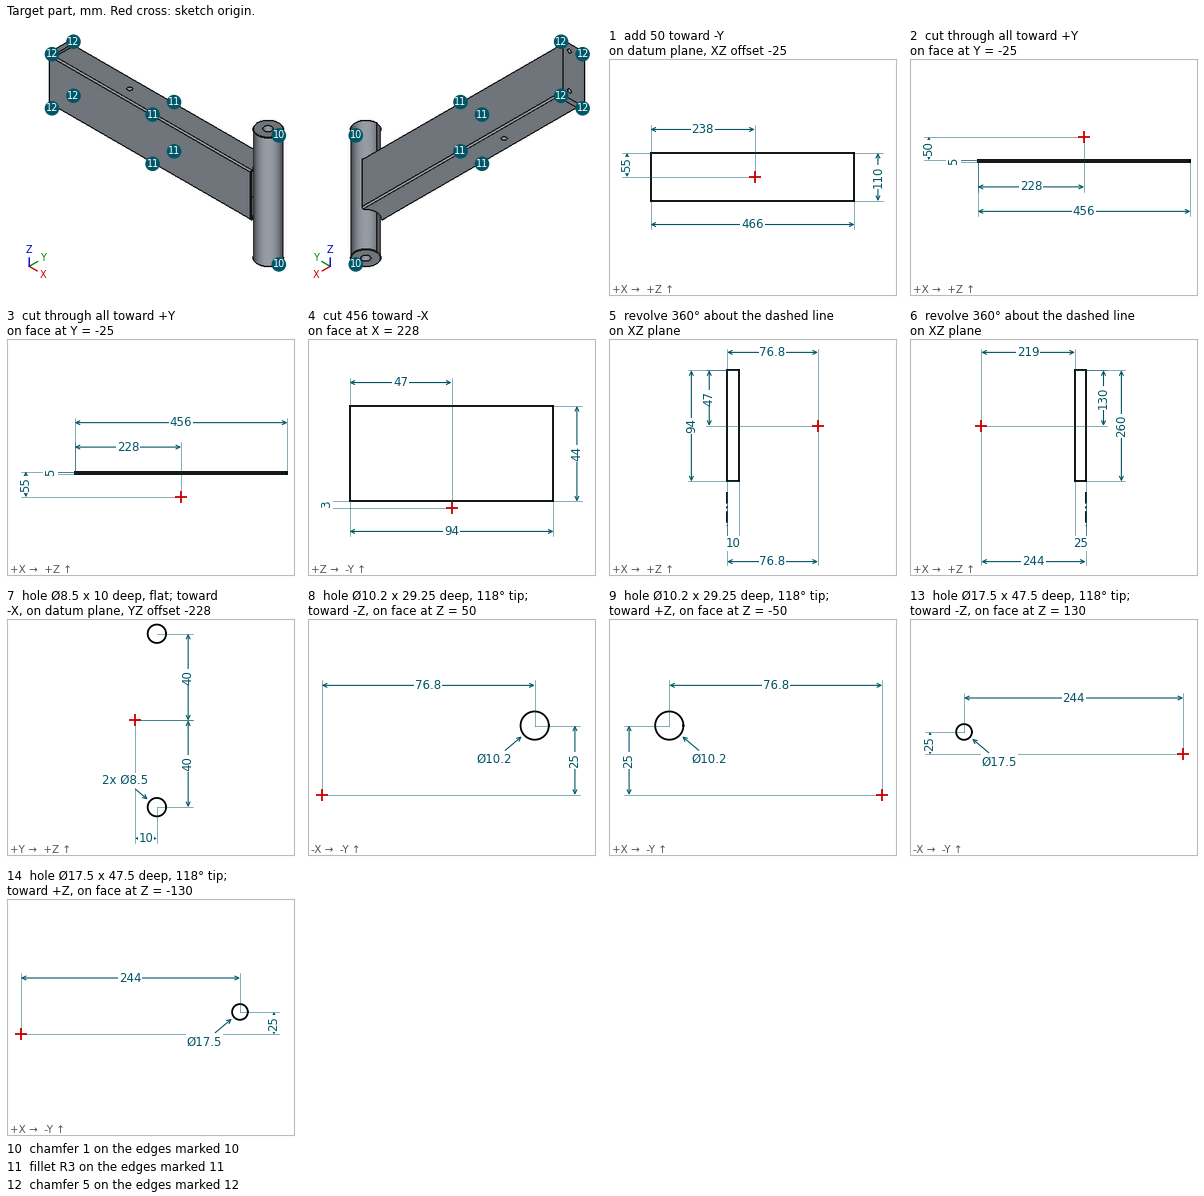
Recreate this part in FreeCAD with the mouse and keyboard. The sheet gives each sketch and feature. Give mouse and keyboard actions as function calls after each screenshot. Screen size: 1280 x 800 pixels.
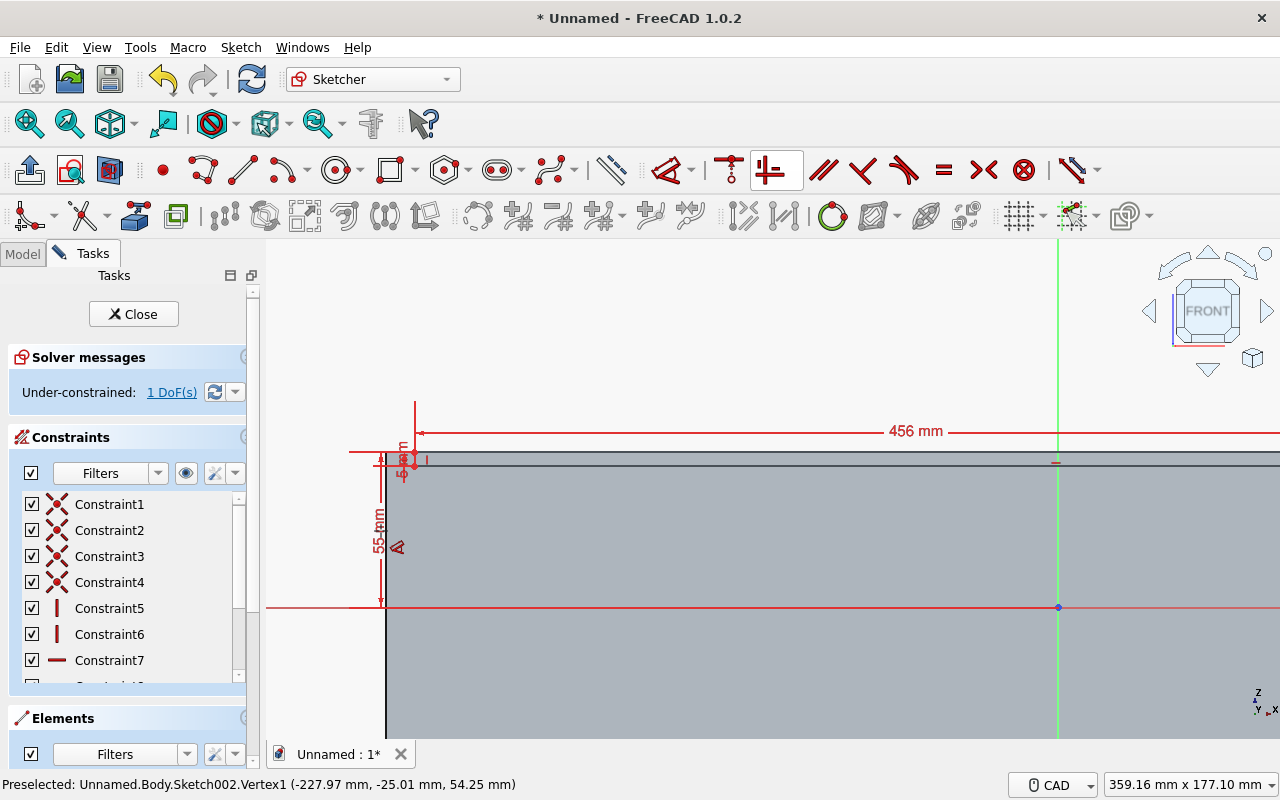
click(415, 452)
click(737, 642)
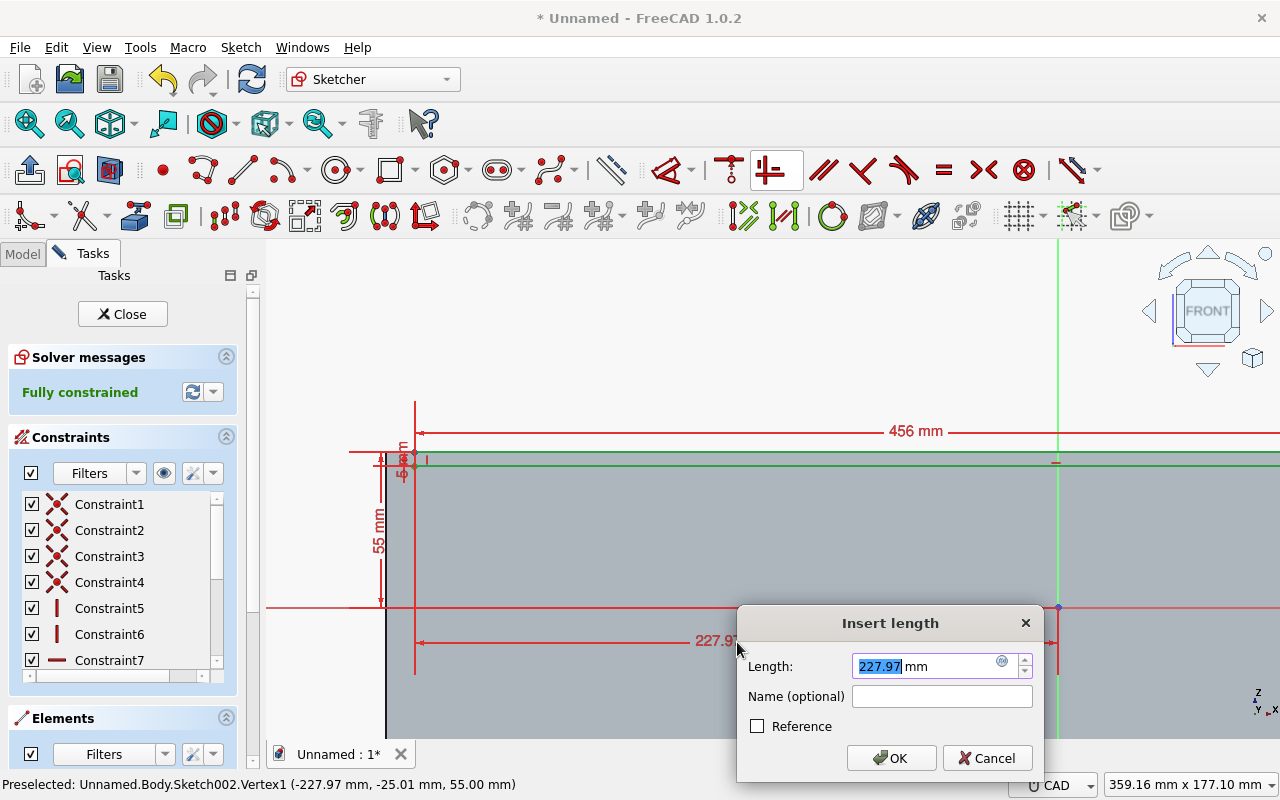
text(228)
key(Return)
key(Escape)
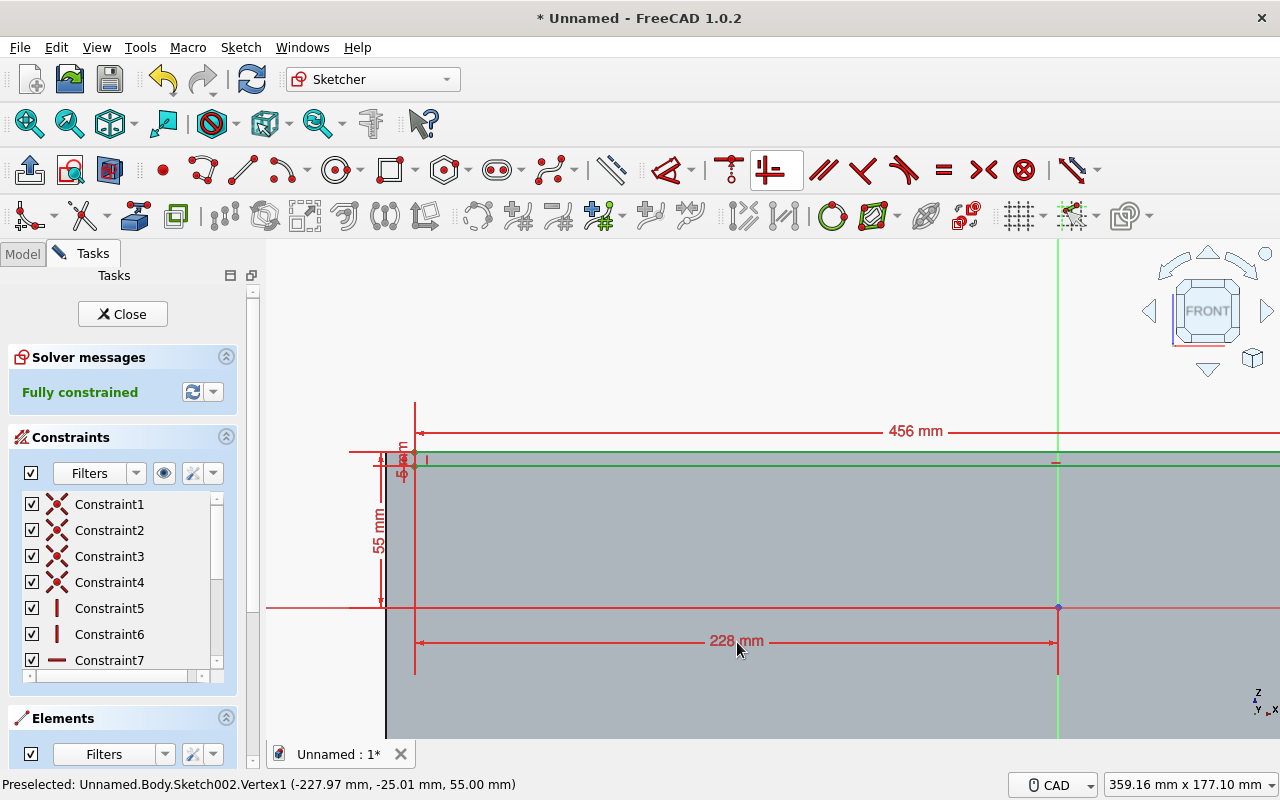
click(123, 314)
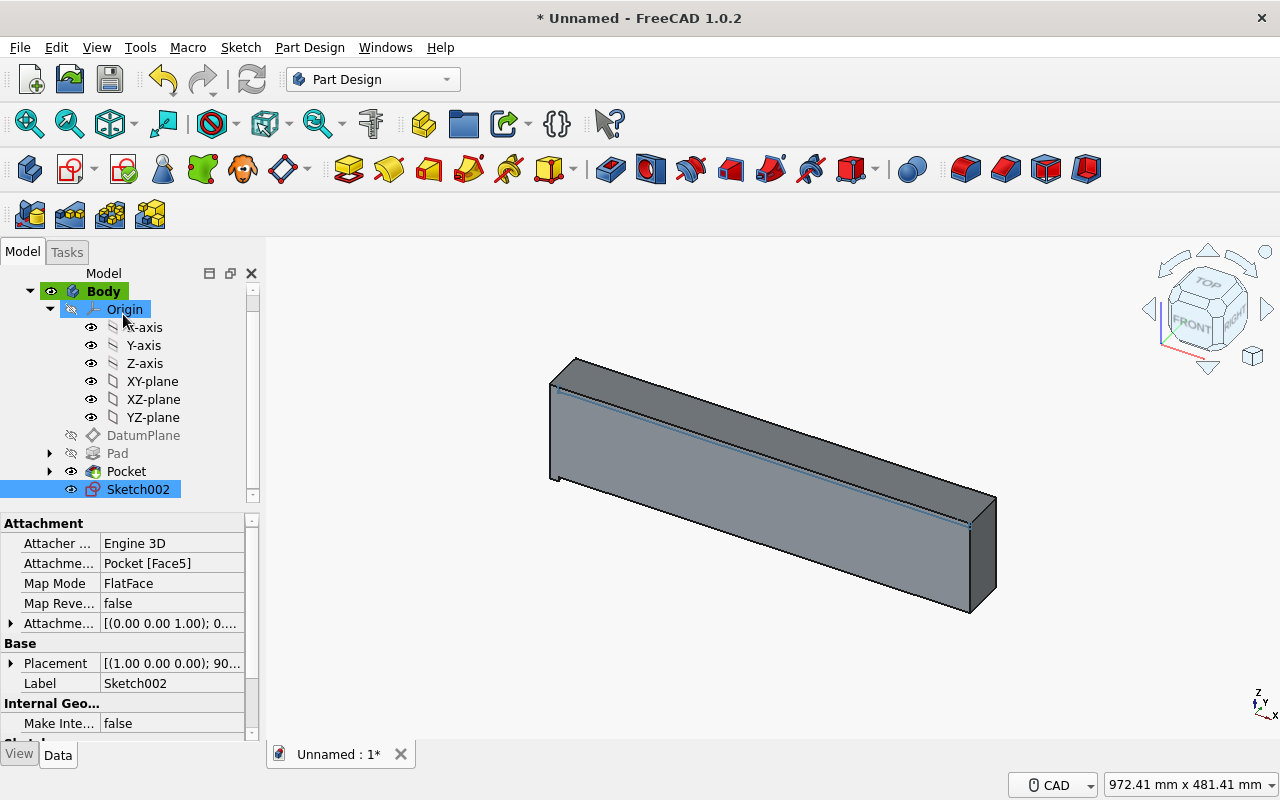
click(612, 170)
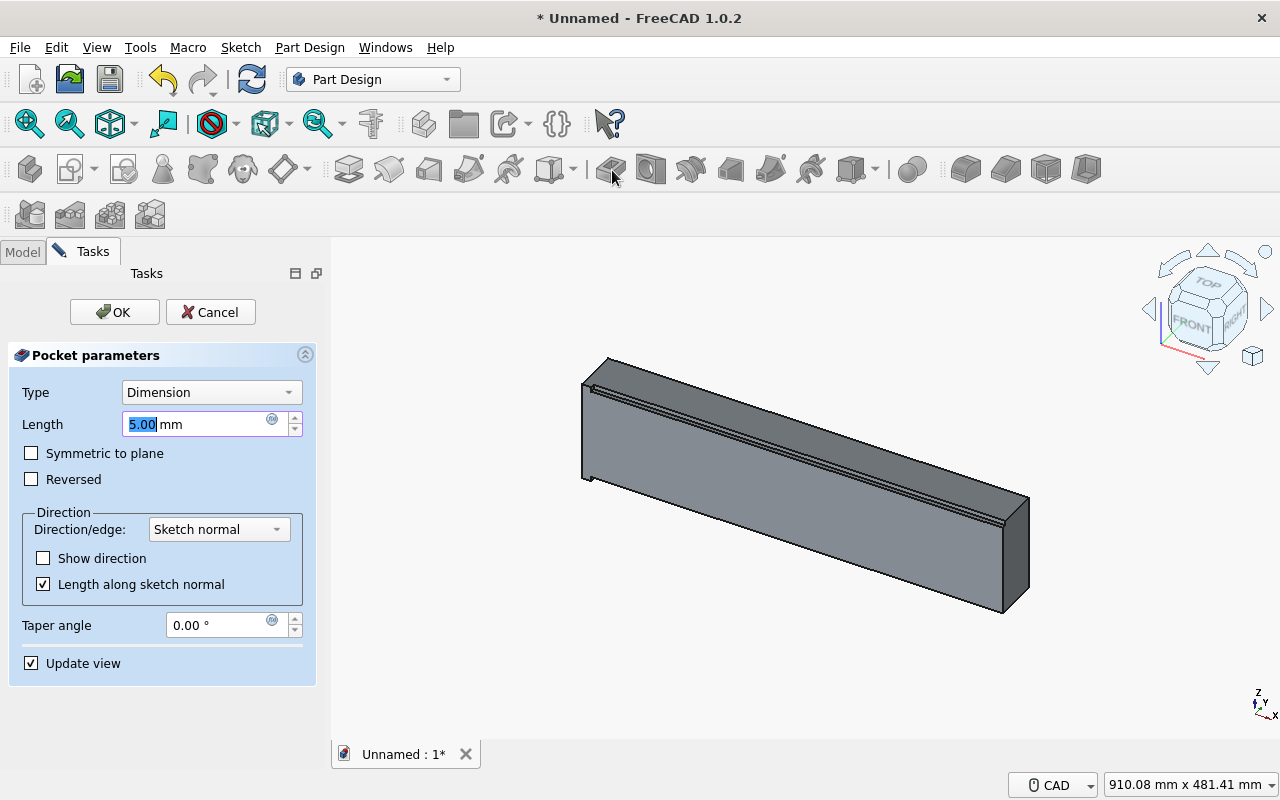
click(212, 392)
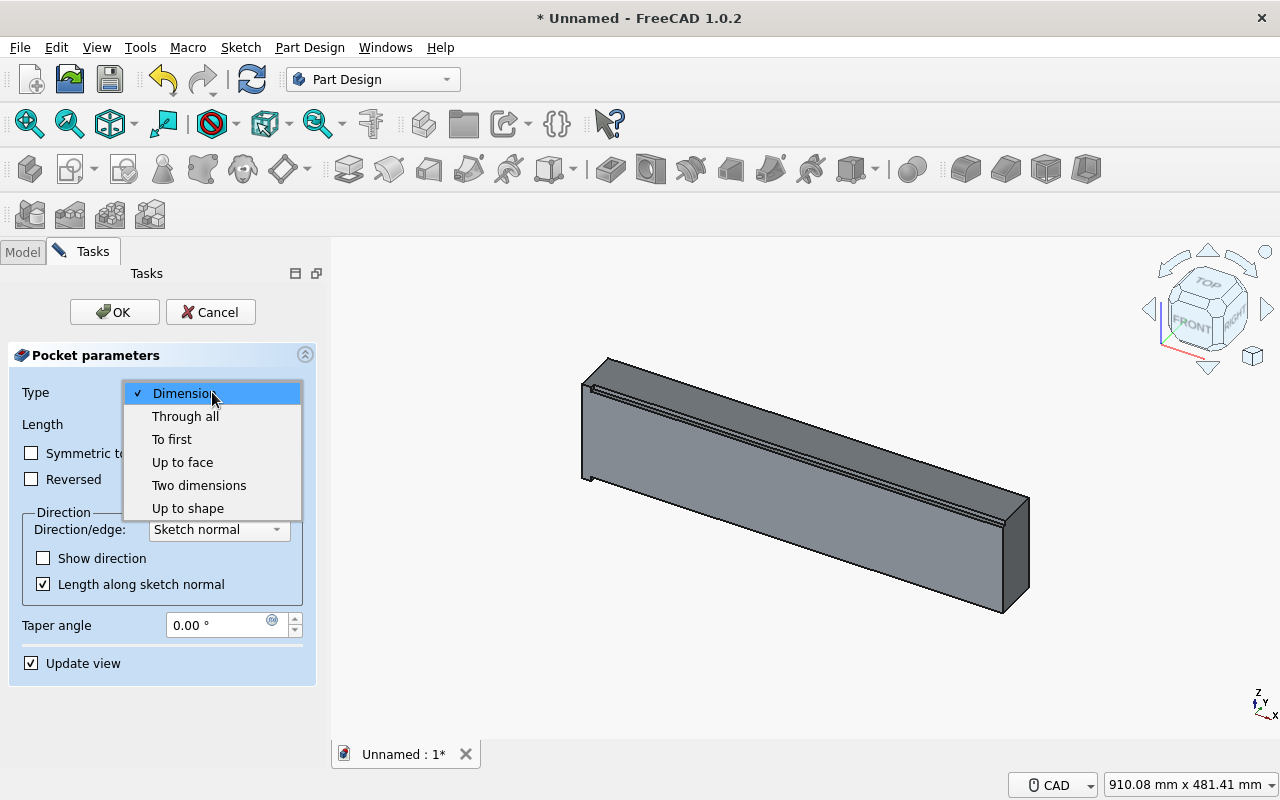
click(212, 416)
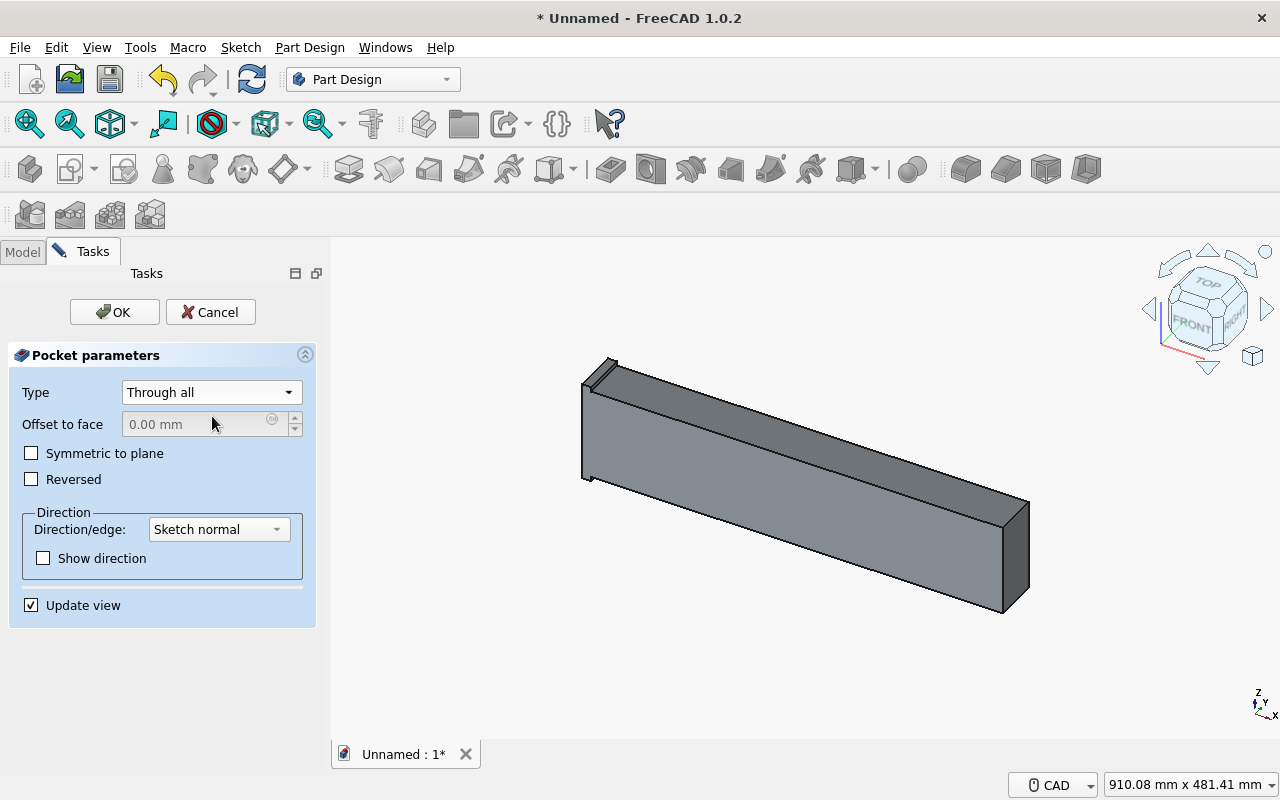
click(115, 312)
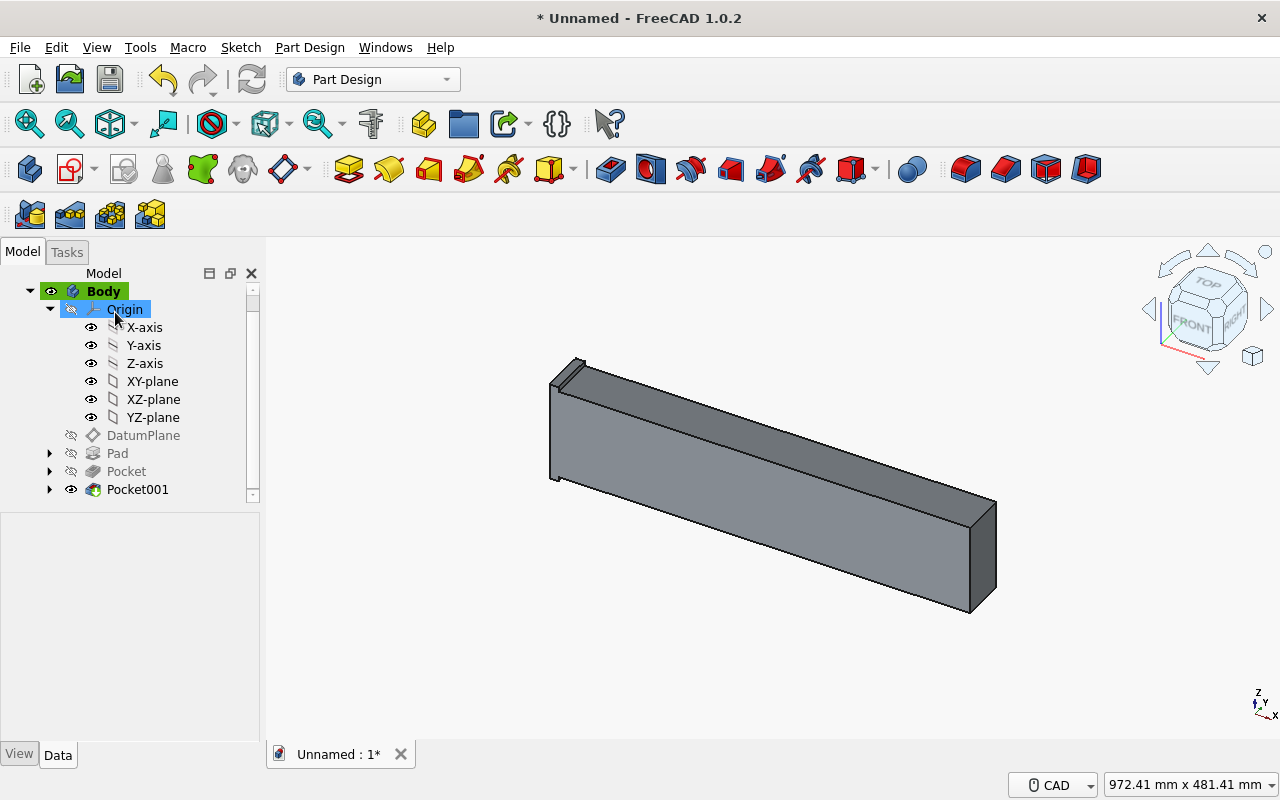
click(983, 544)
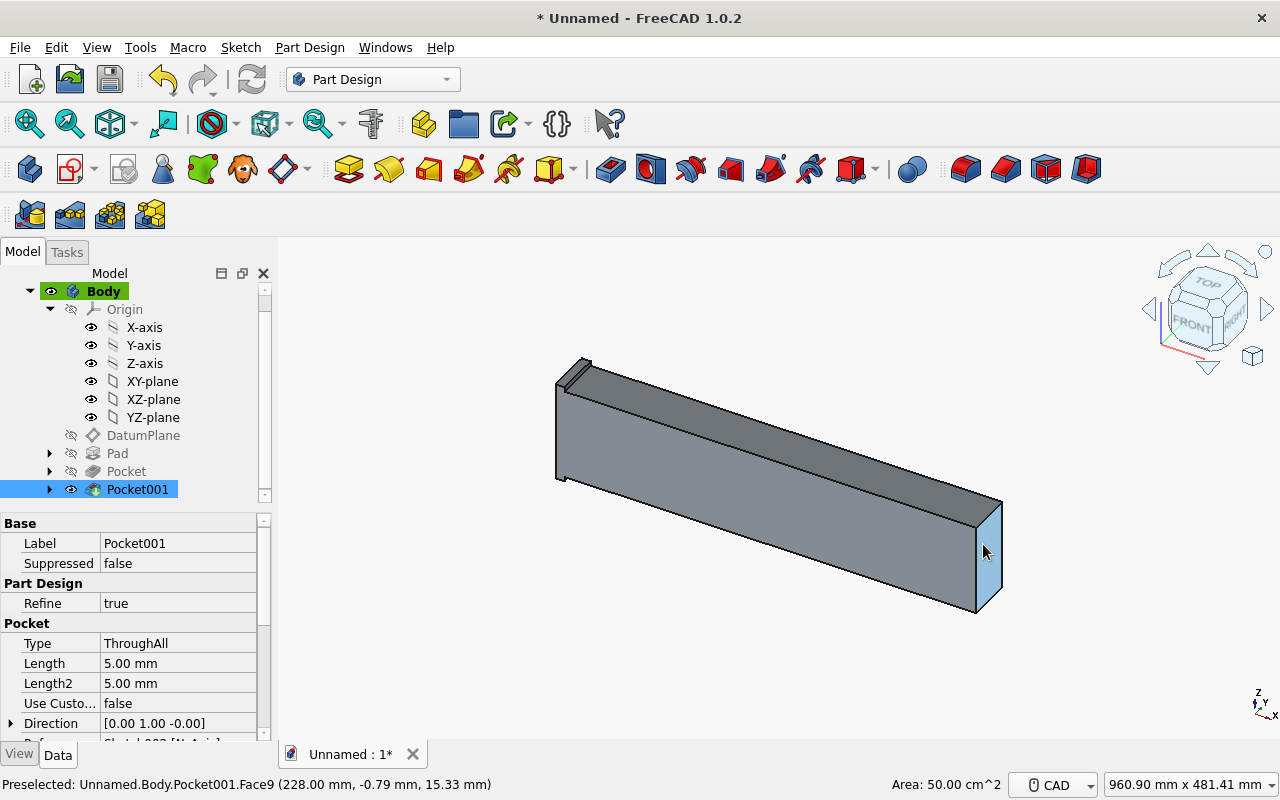
click(70, 170)